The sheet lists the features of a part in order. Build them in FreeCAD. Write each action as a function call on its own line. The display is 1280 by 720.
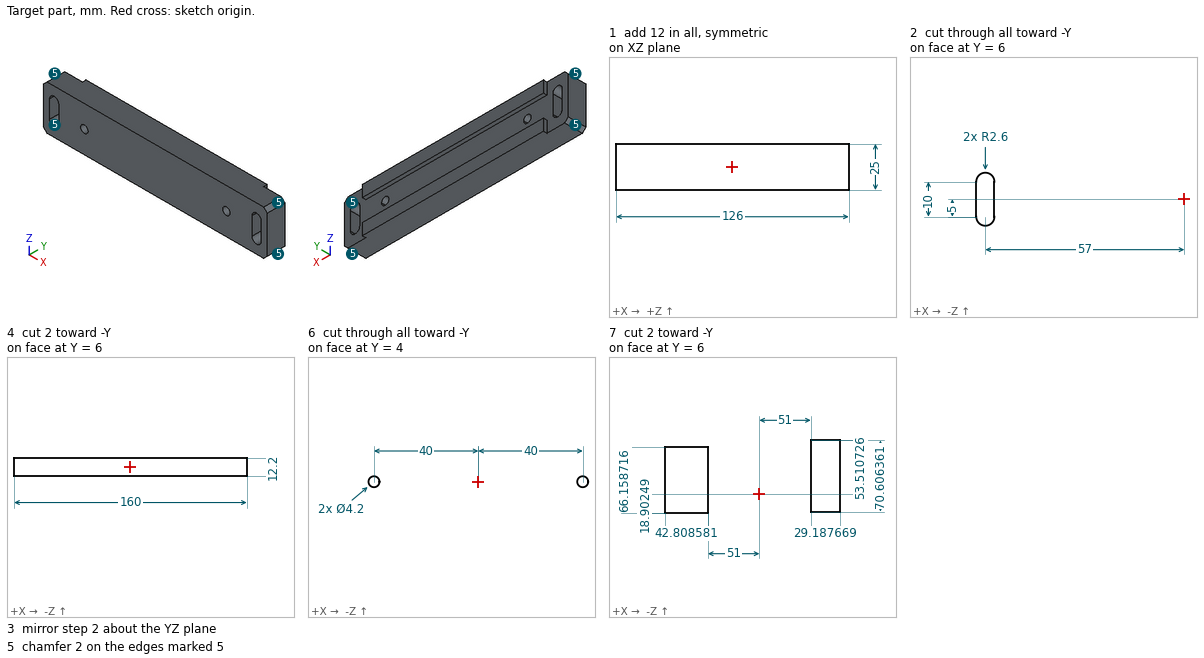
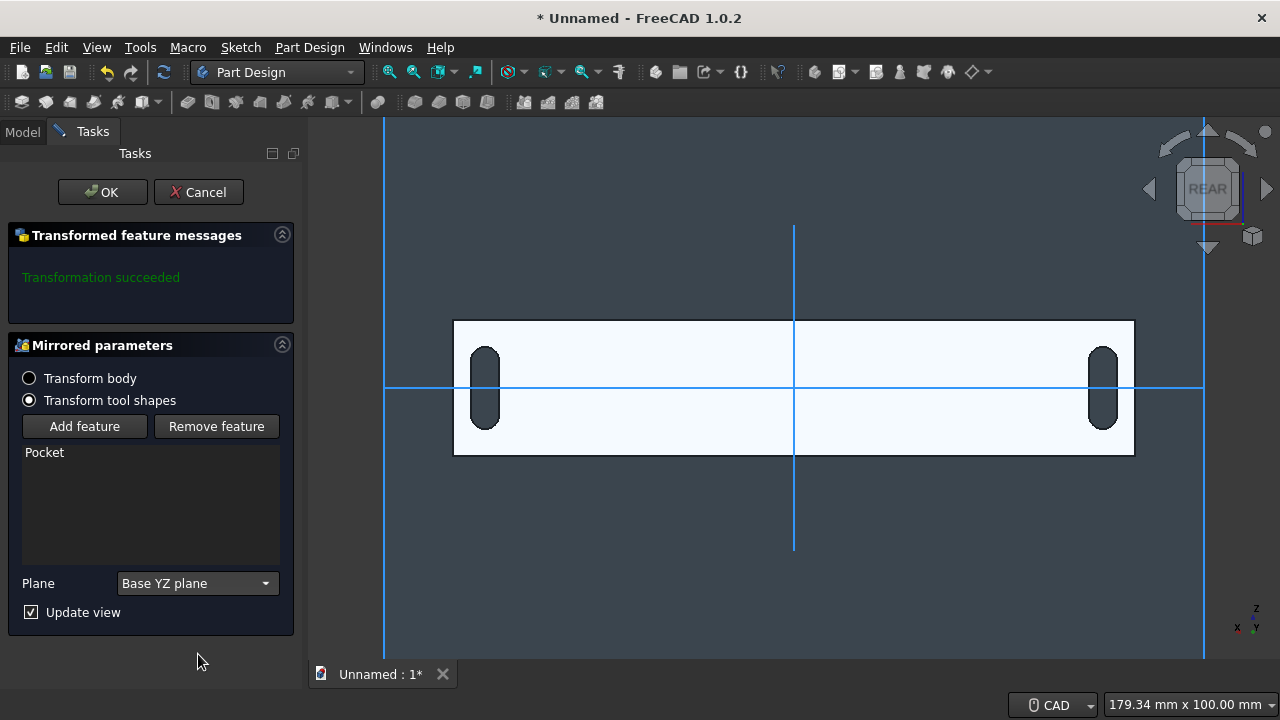
click(103, 192)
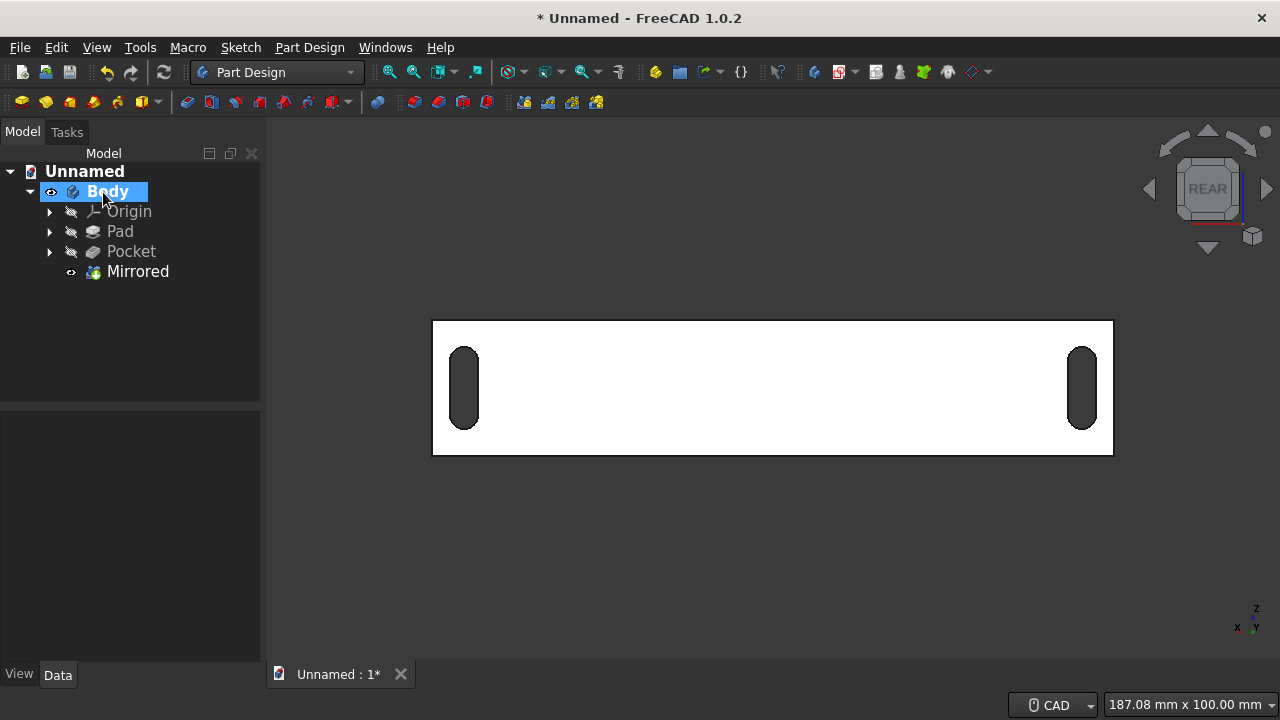
click(578, 387)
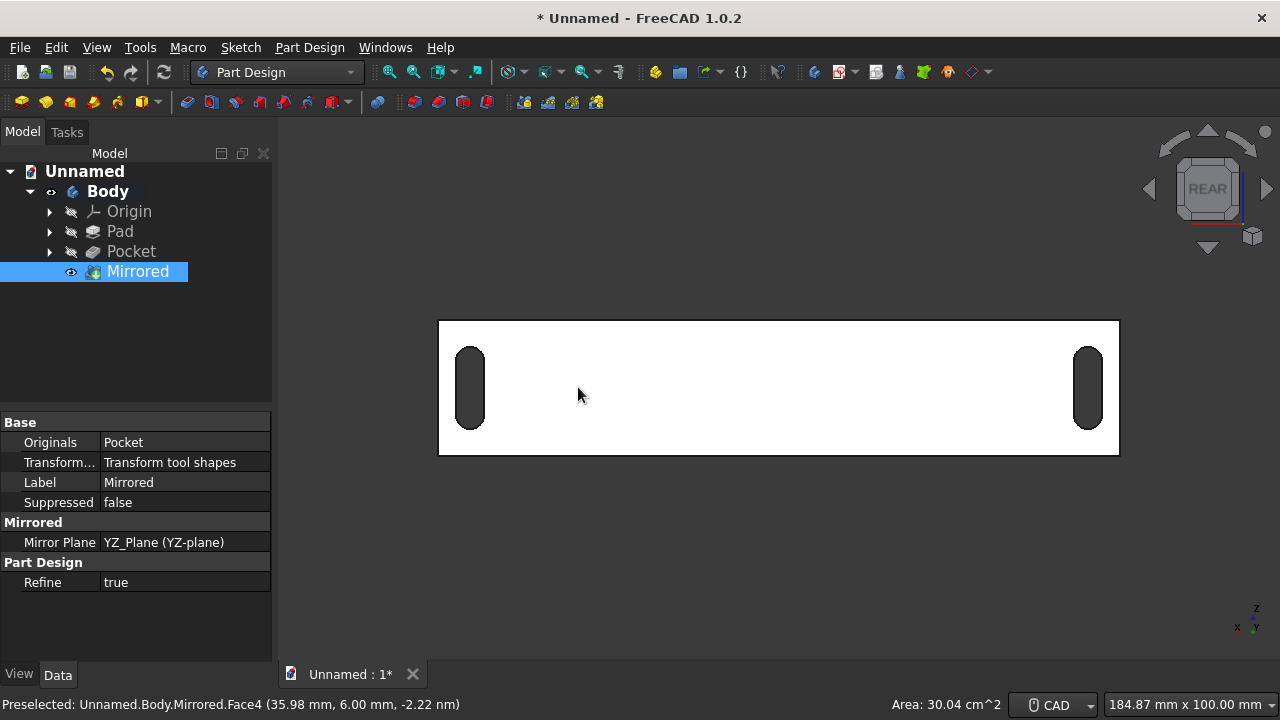
click(840, 72)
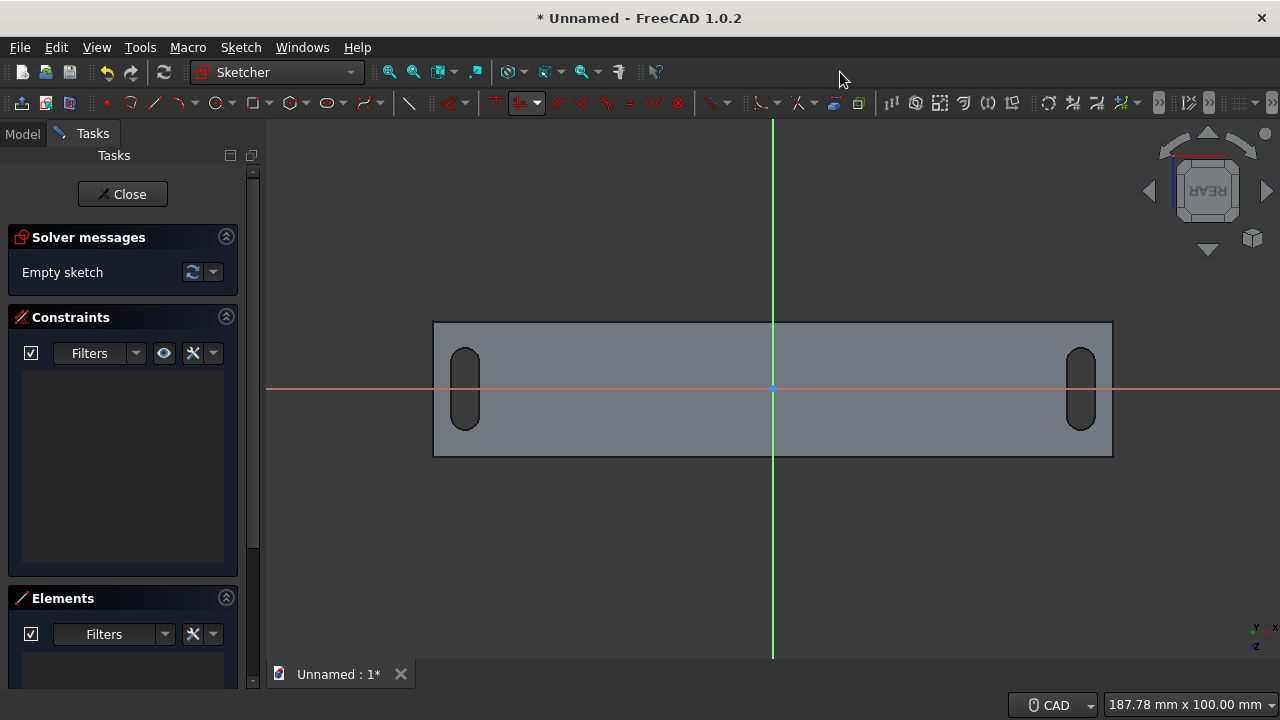
scroll(565, 389, down, 2)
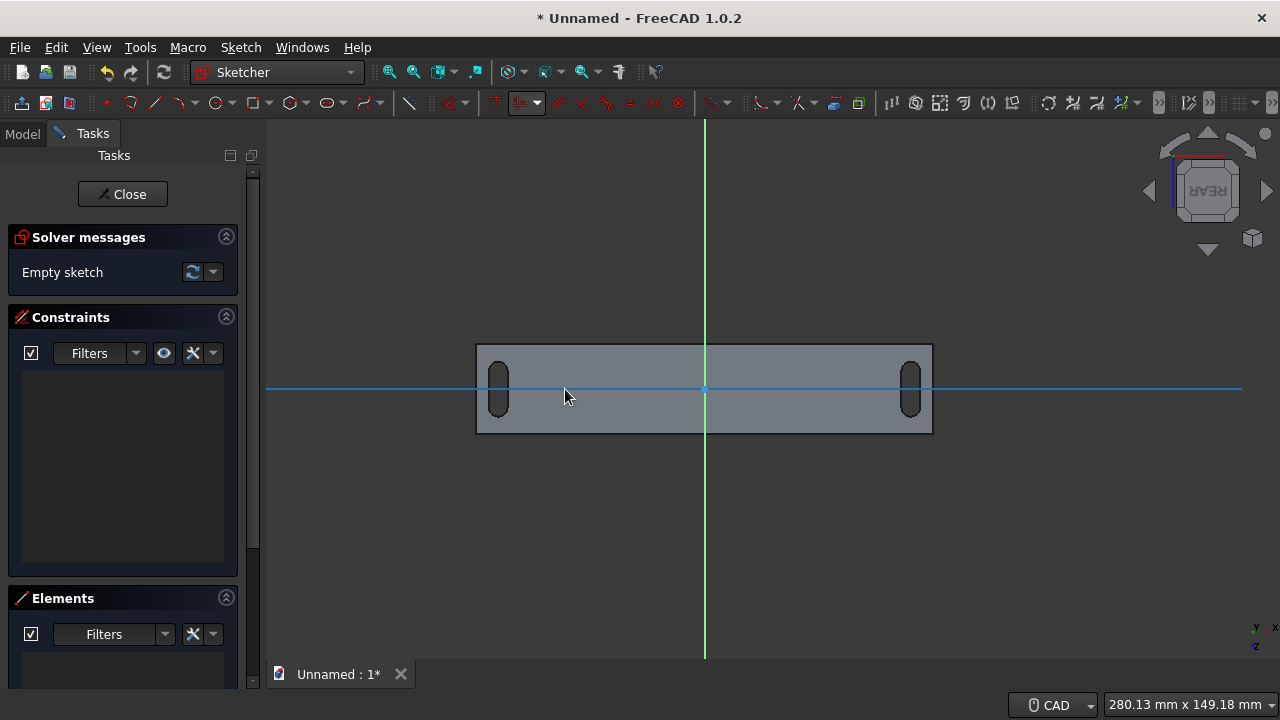
key(g)
key(v)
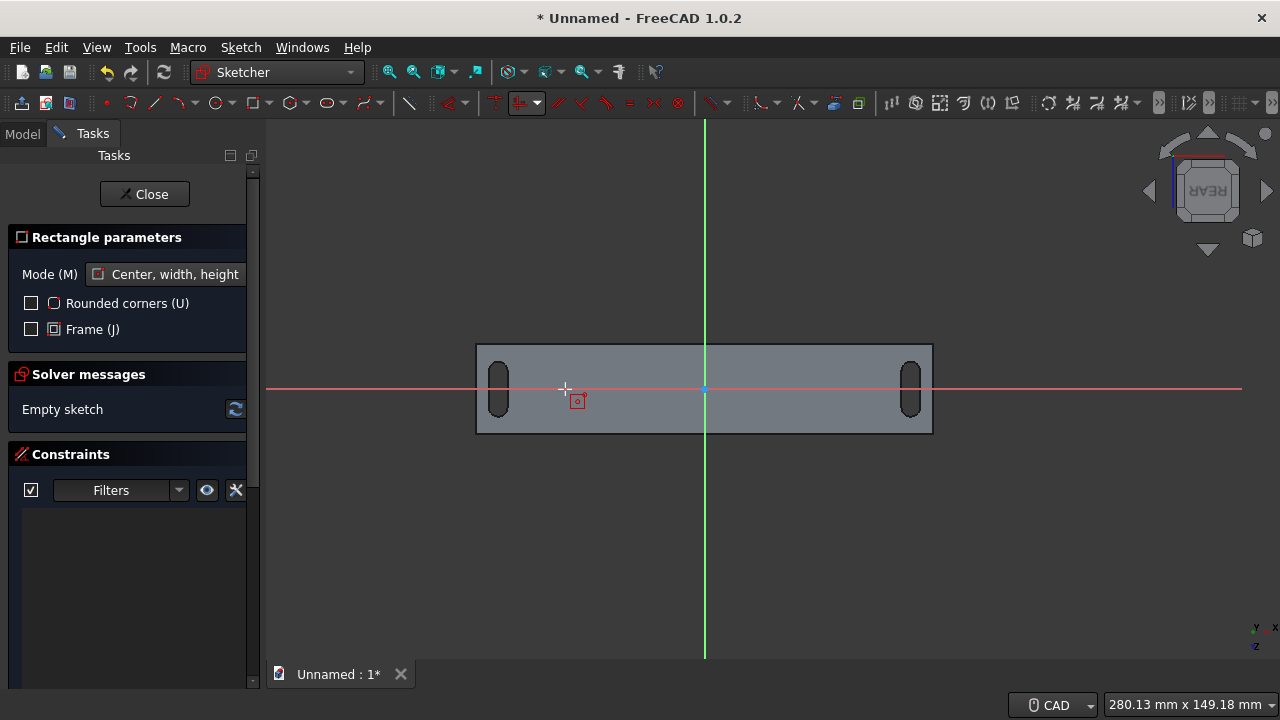
click(705, 389)
click(994, 367)
key(Escape)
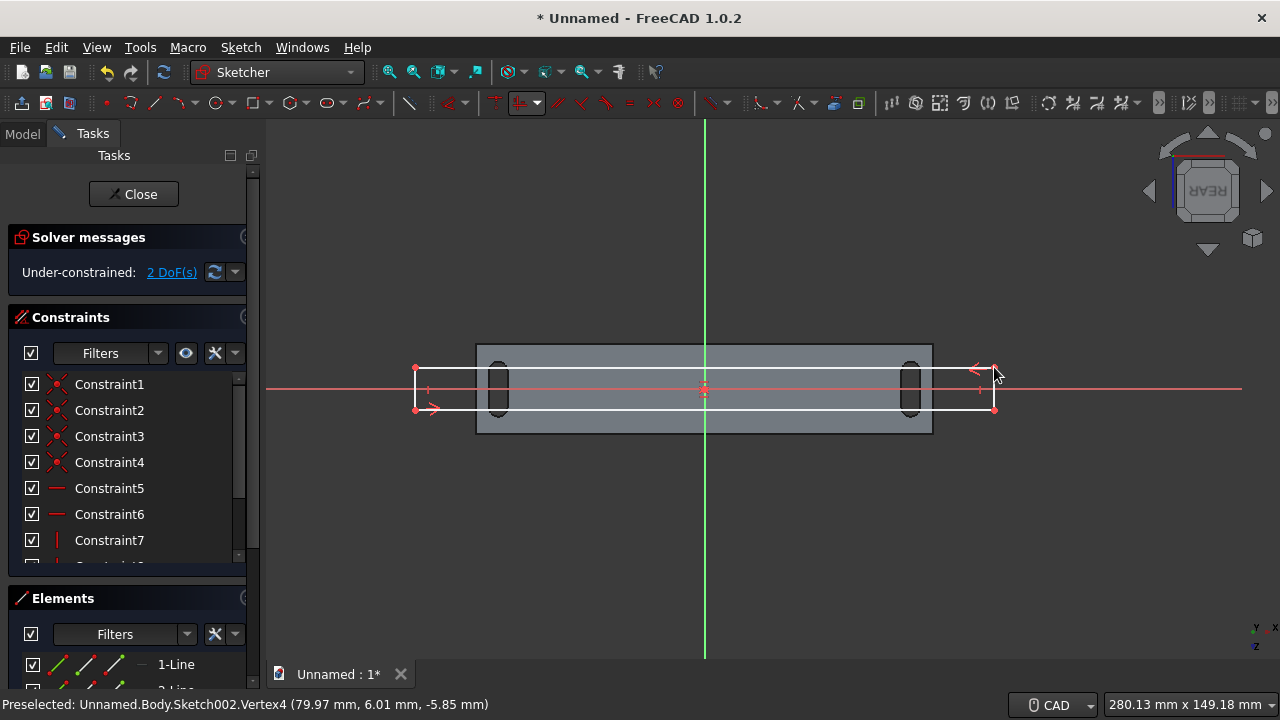
click(448, 104)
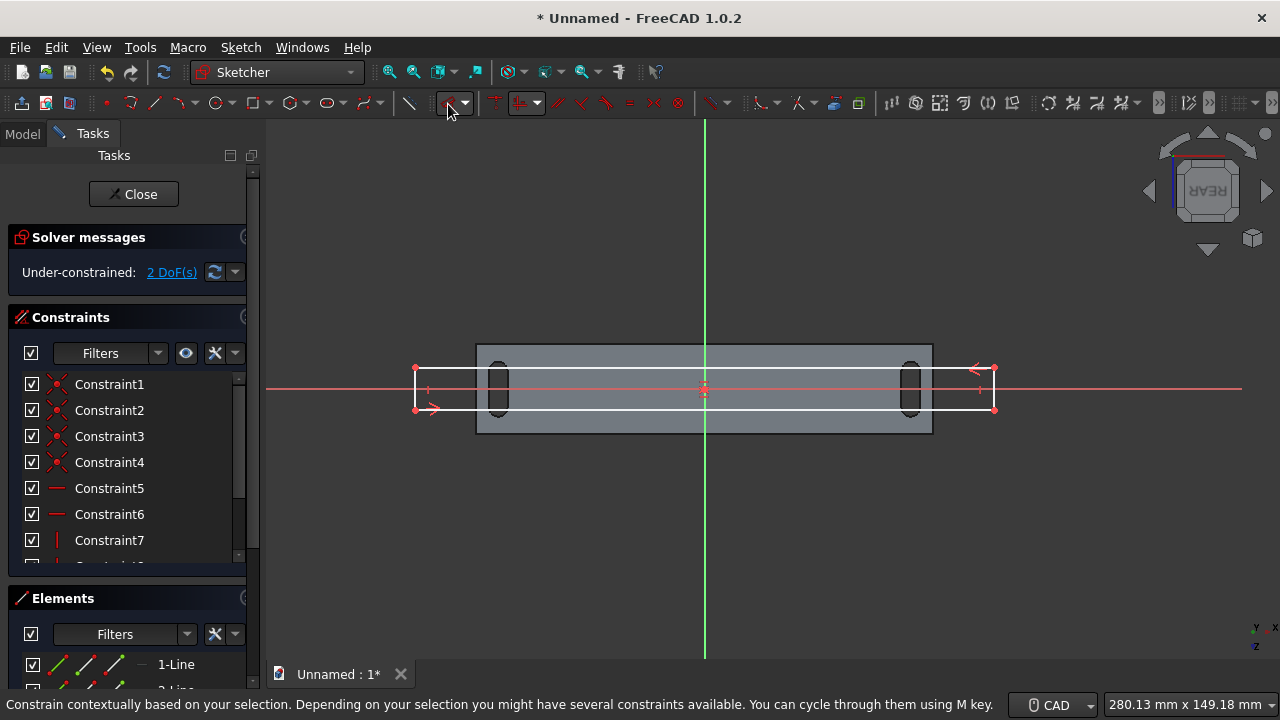
click(589, 410)
click(571, 444)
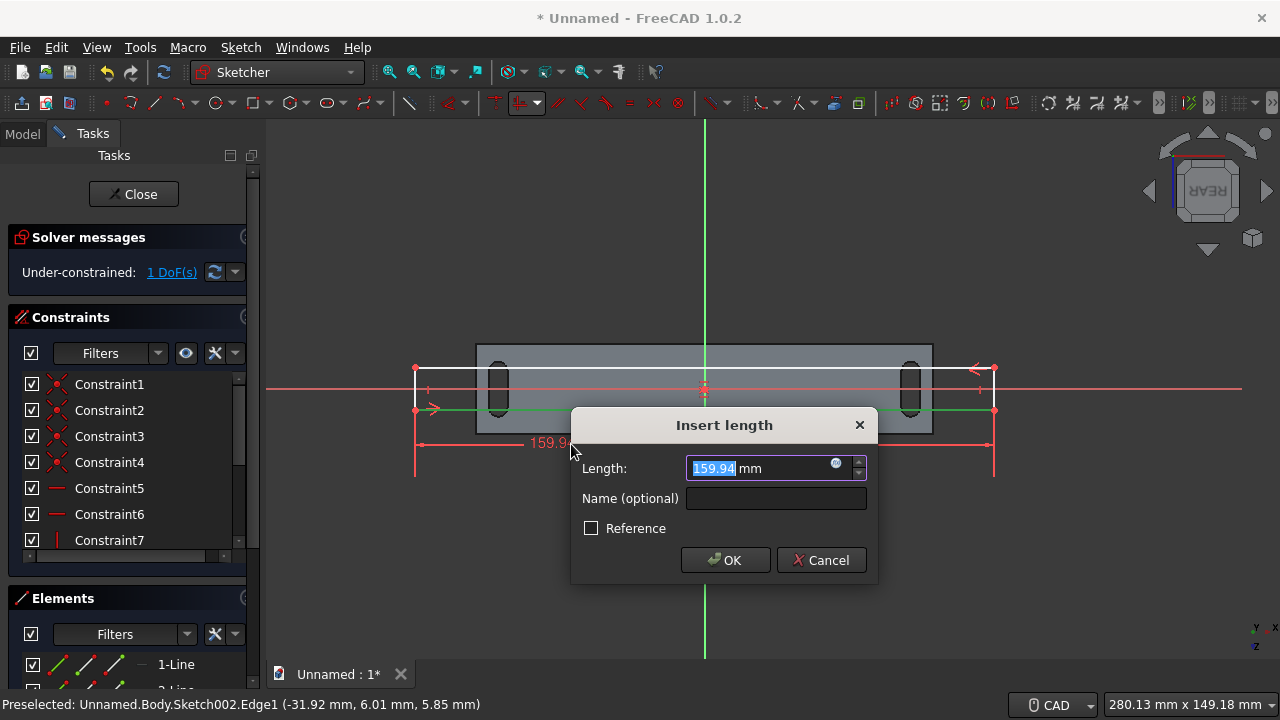
text(160)
key(Return)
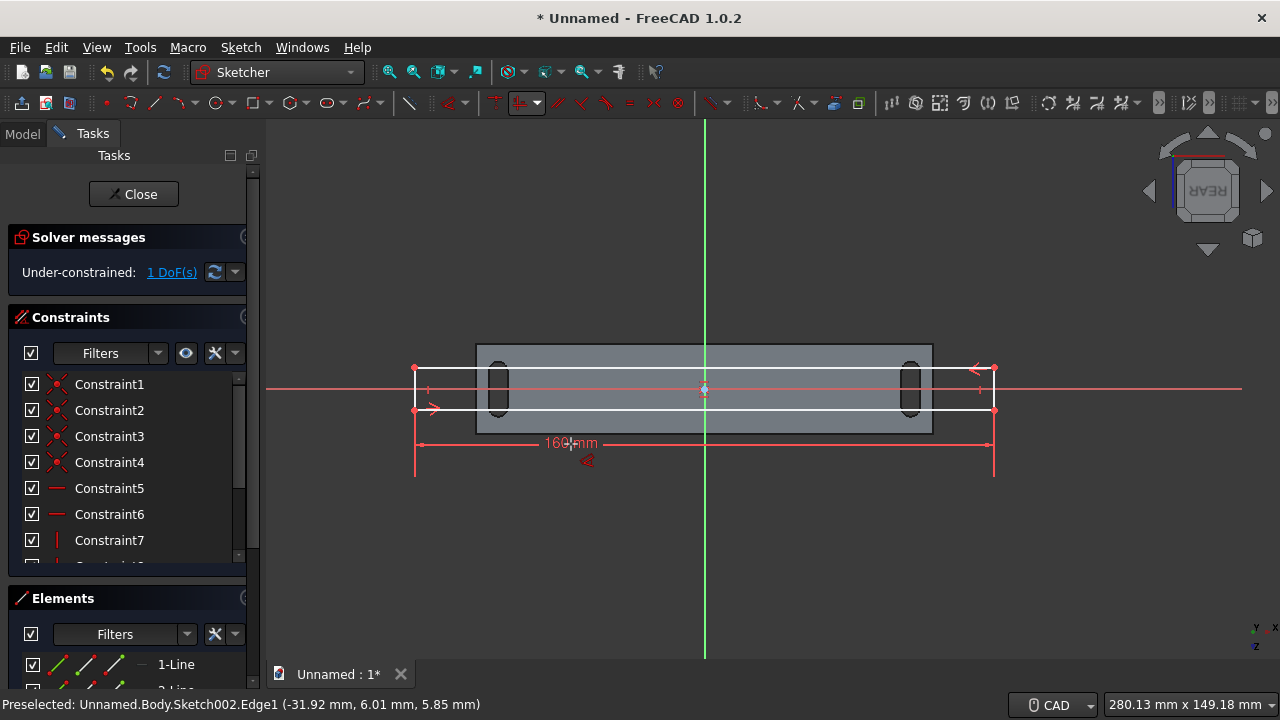
click(994, 389)
click(1028, 374)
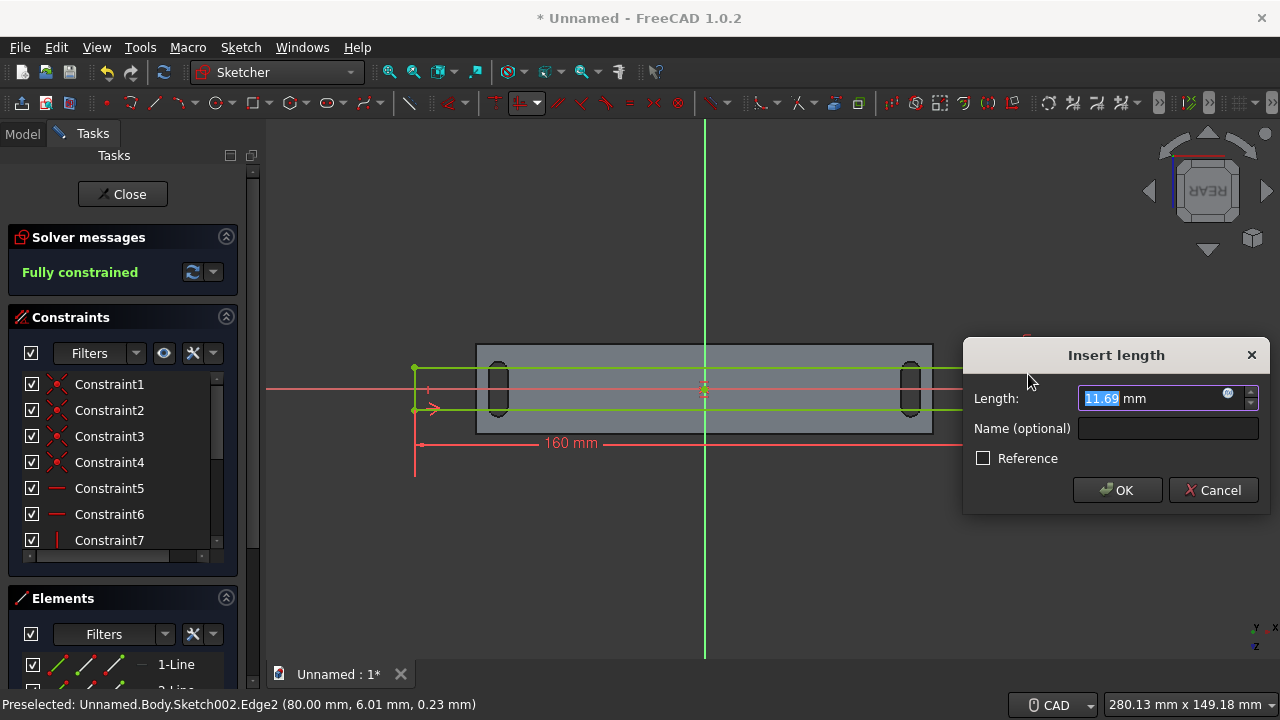
text(12.2)
key(Return)
key(Escape)